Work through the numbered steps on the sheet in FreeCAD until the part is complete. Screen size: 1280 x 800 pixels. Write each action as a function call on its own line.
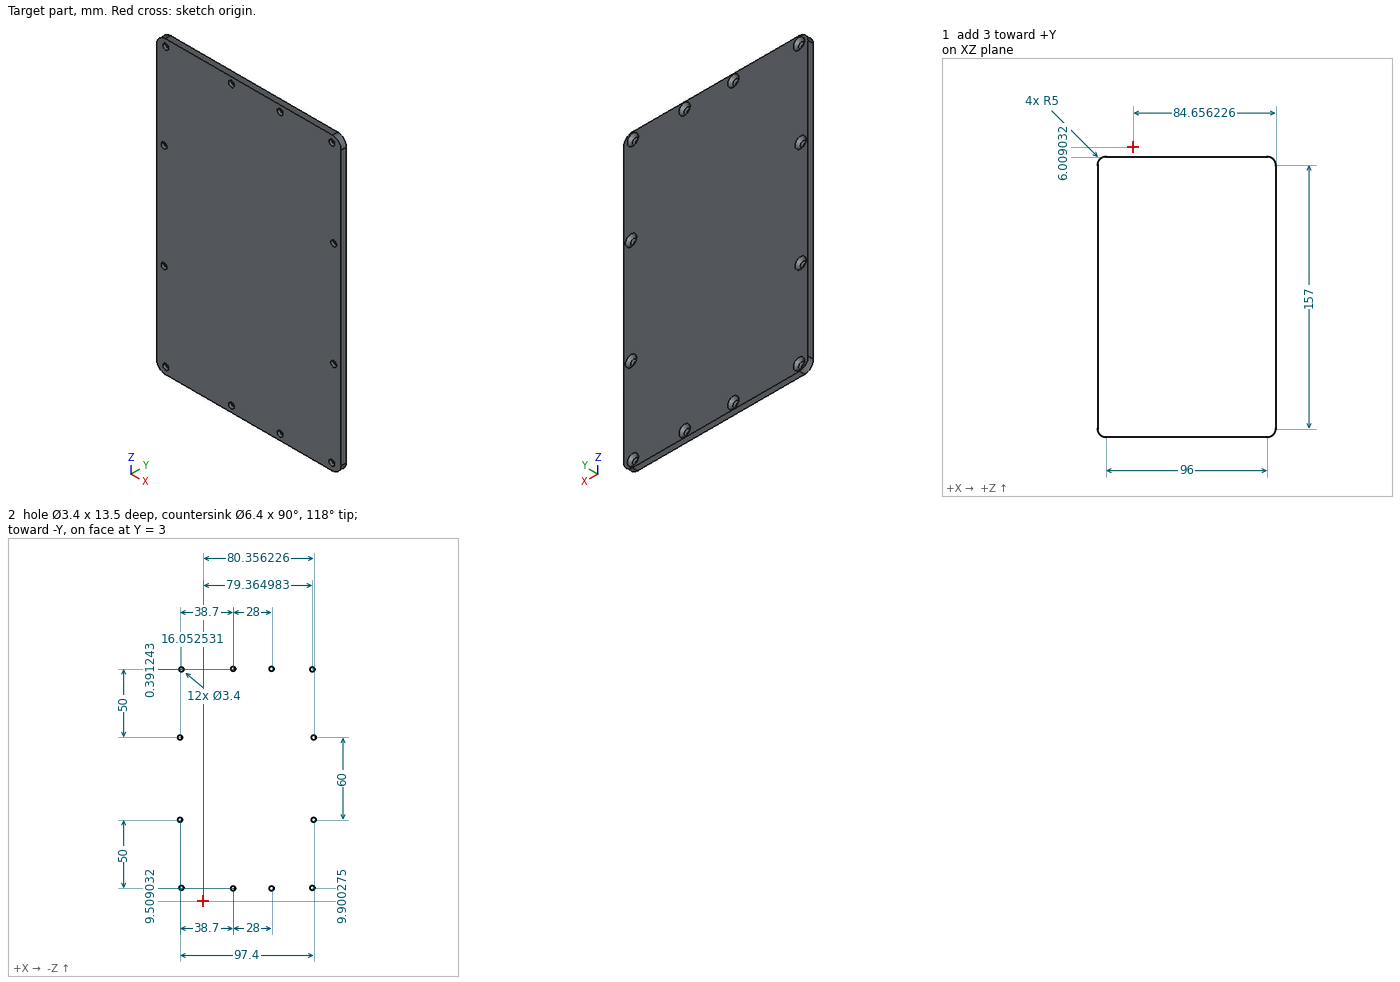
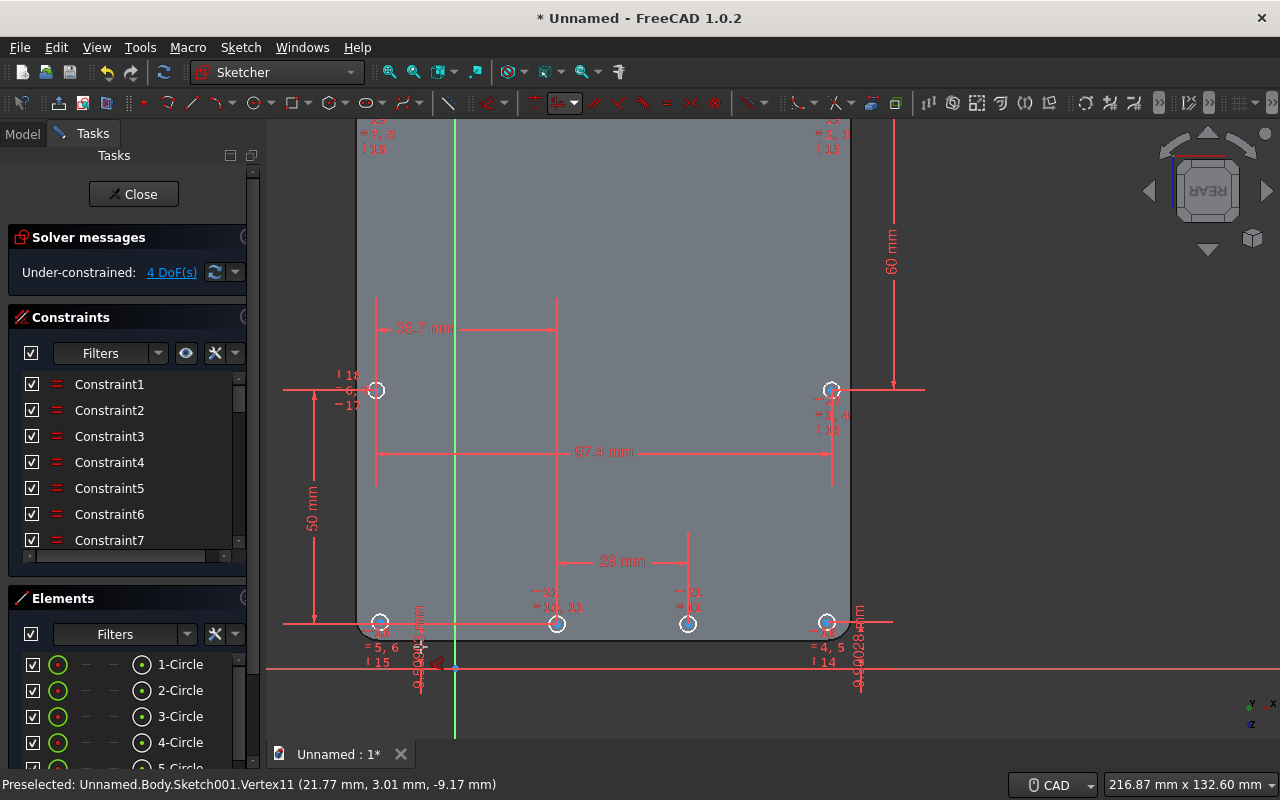
scroll(827, 624, down, 3)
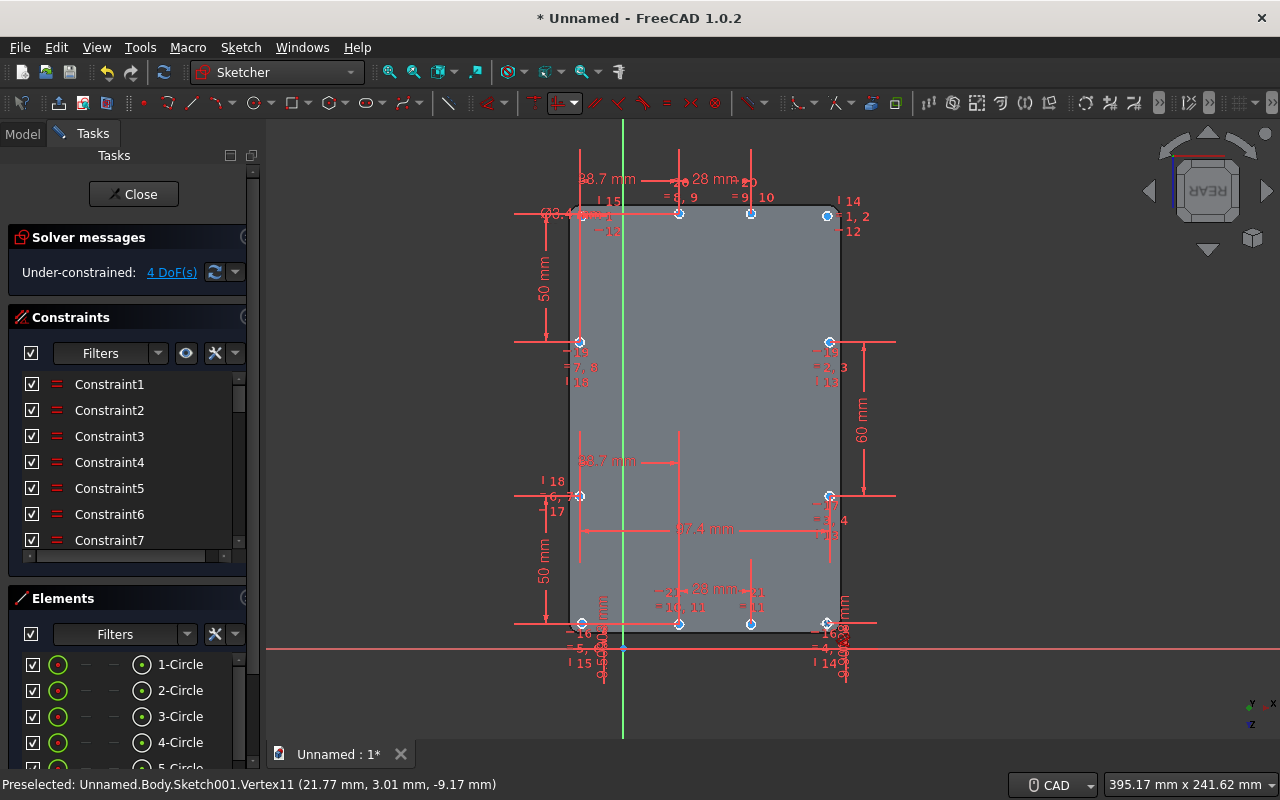
click(582, 216)
click(603, 683)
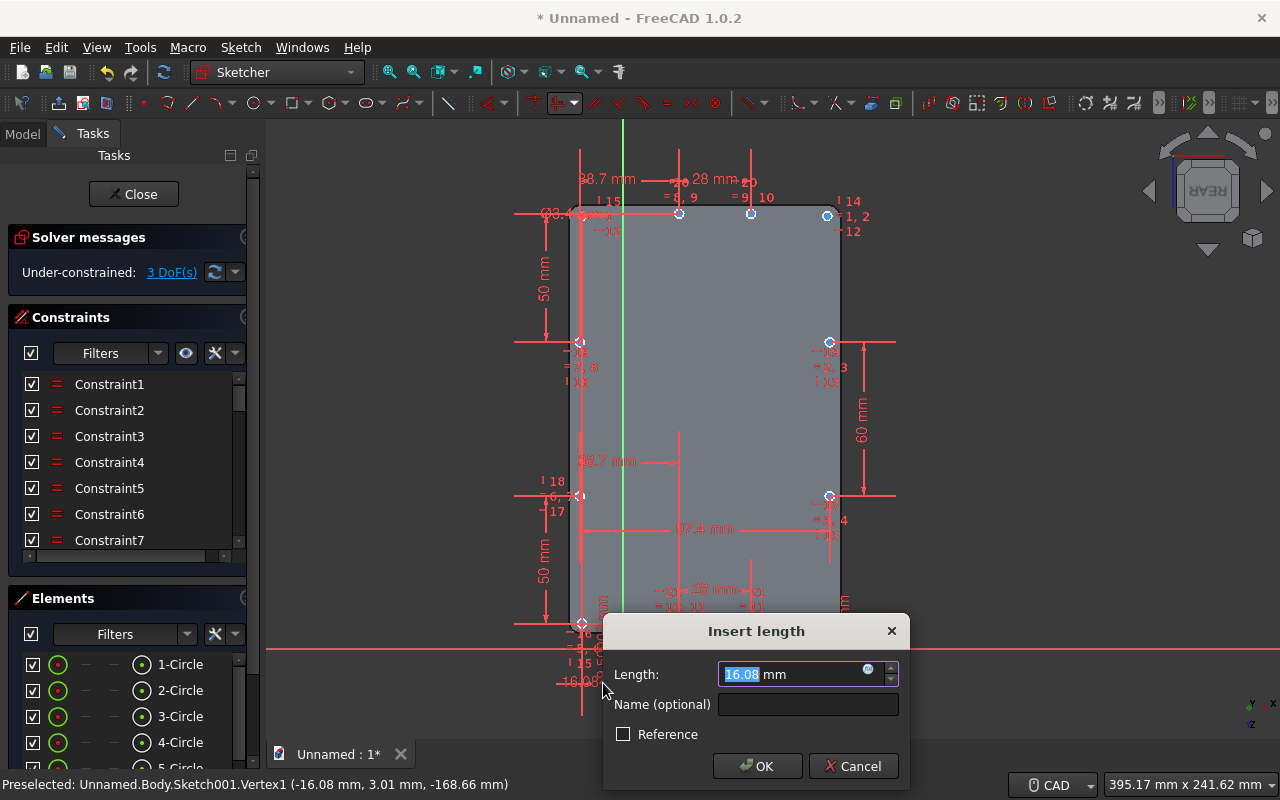
text(16.052531)
key(Return)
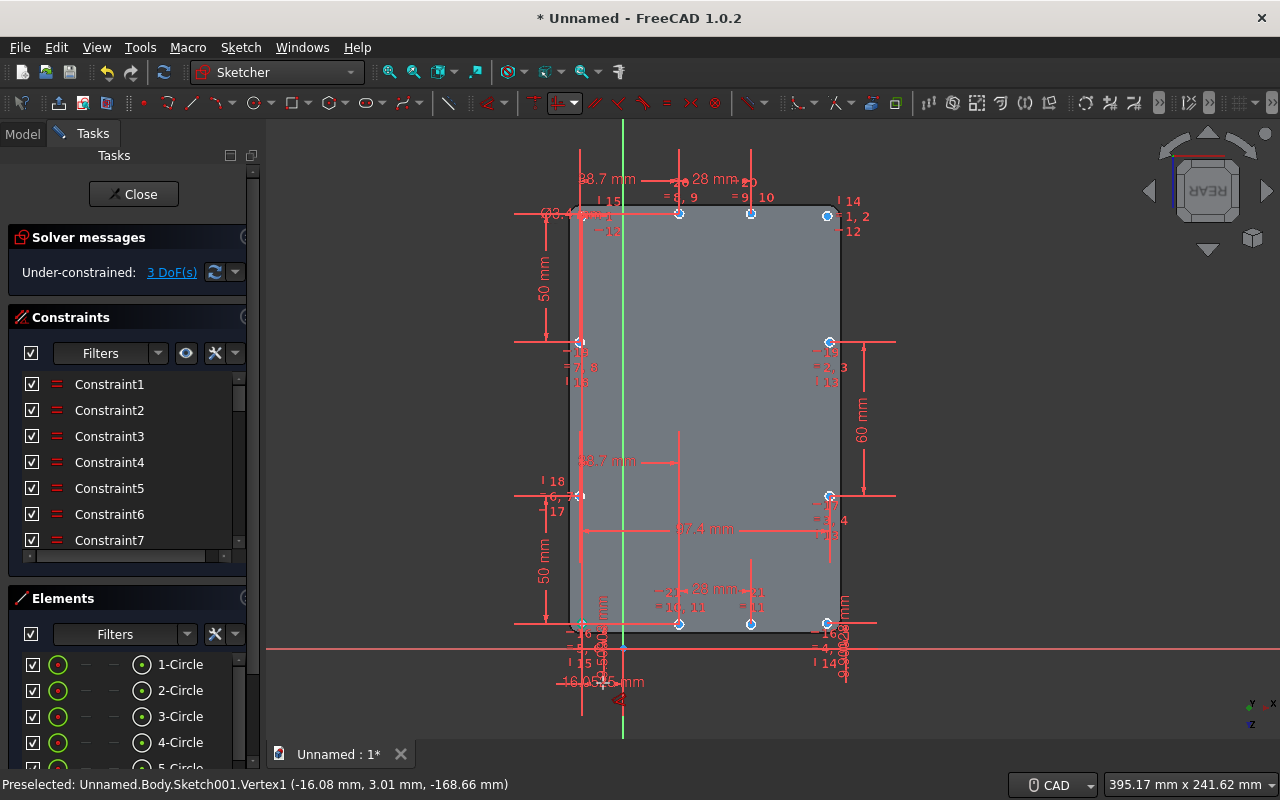
click(827, 216)
click(725, 683)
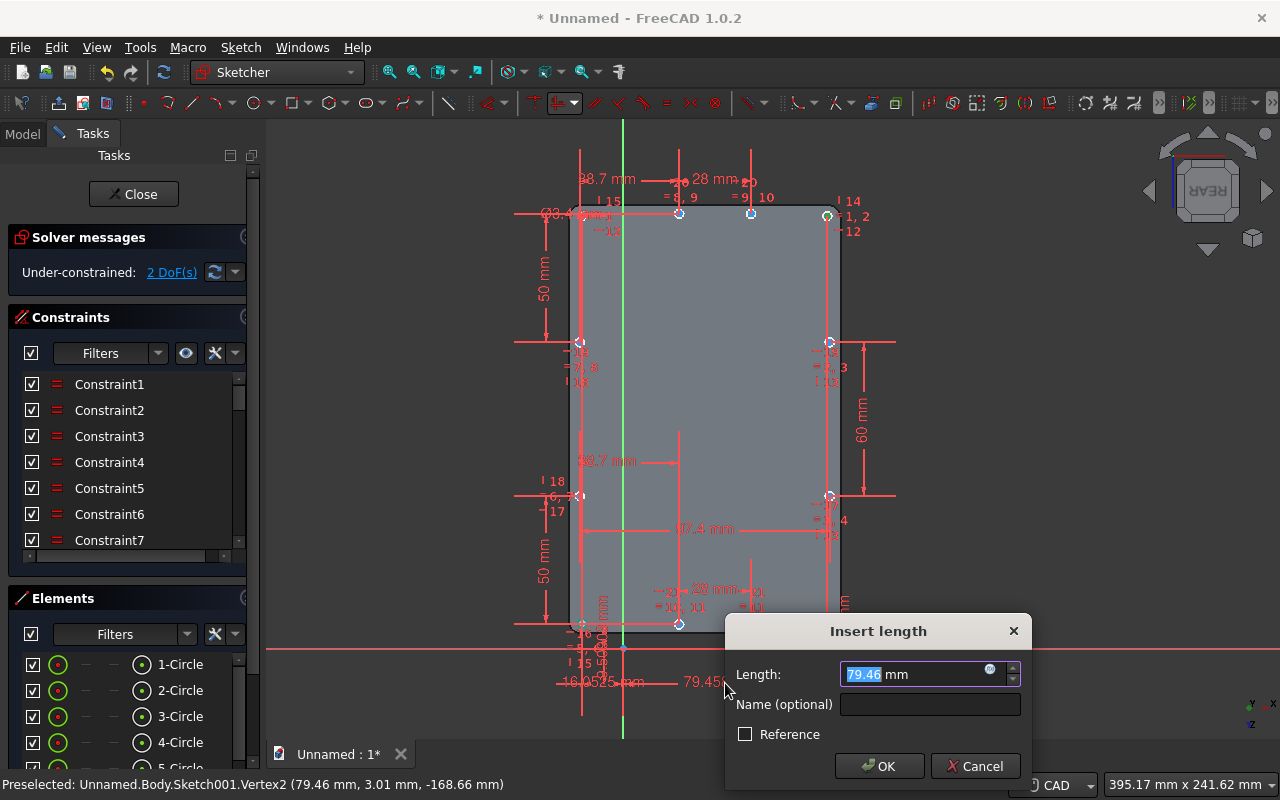
text(79.364983)
key(Return)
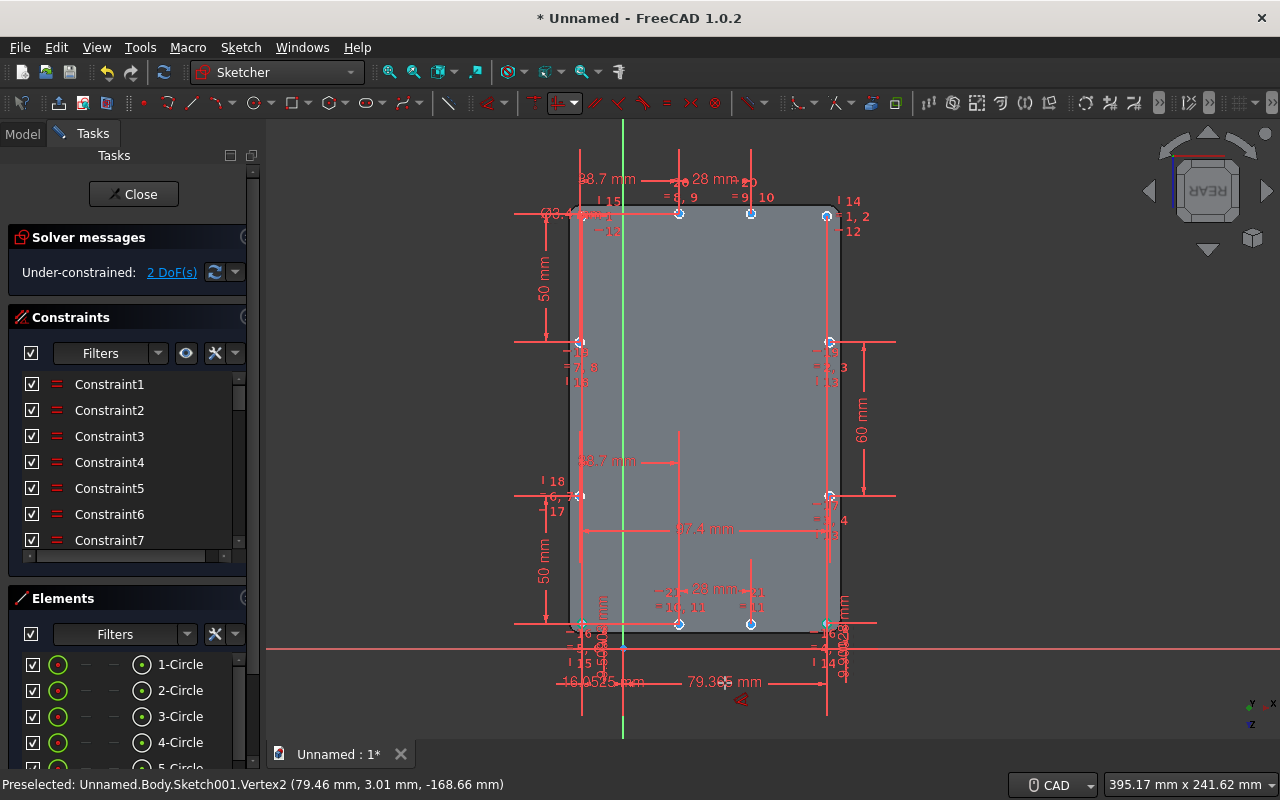
click(830, 342)
click(799, 683)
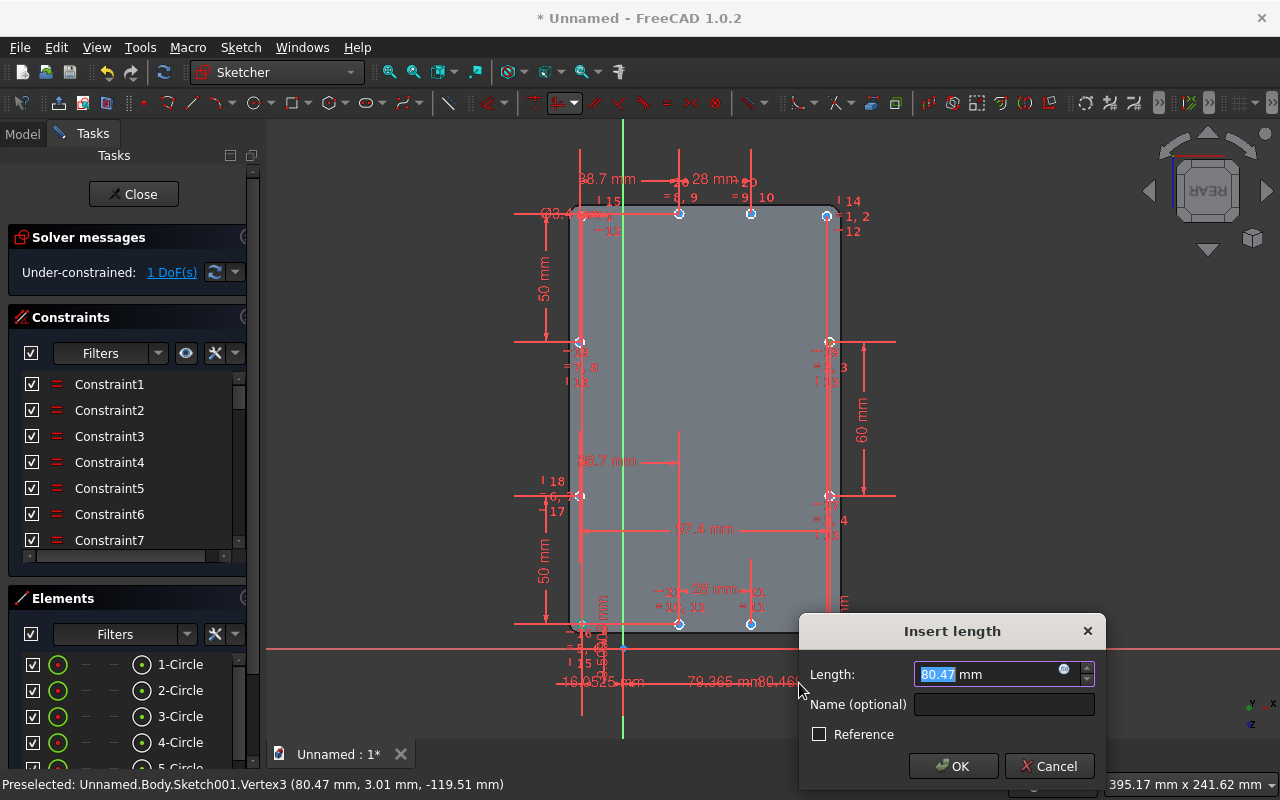
text(80.356226)
key(Return)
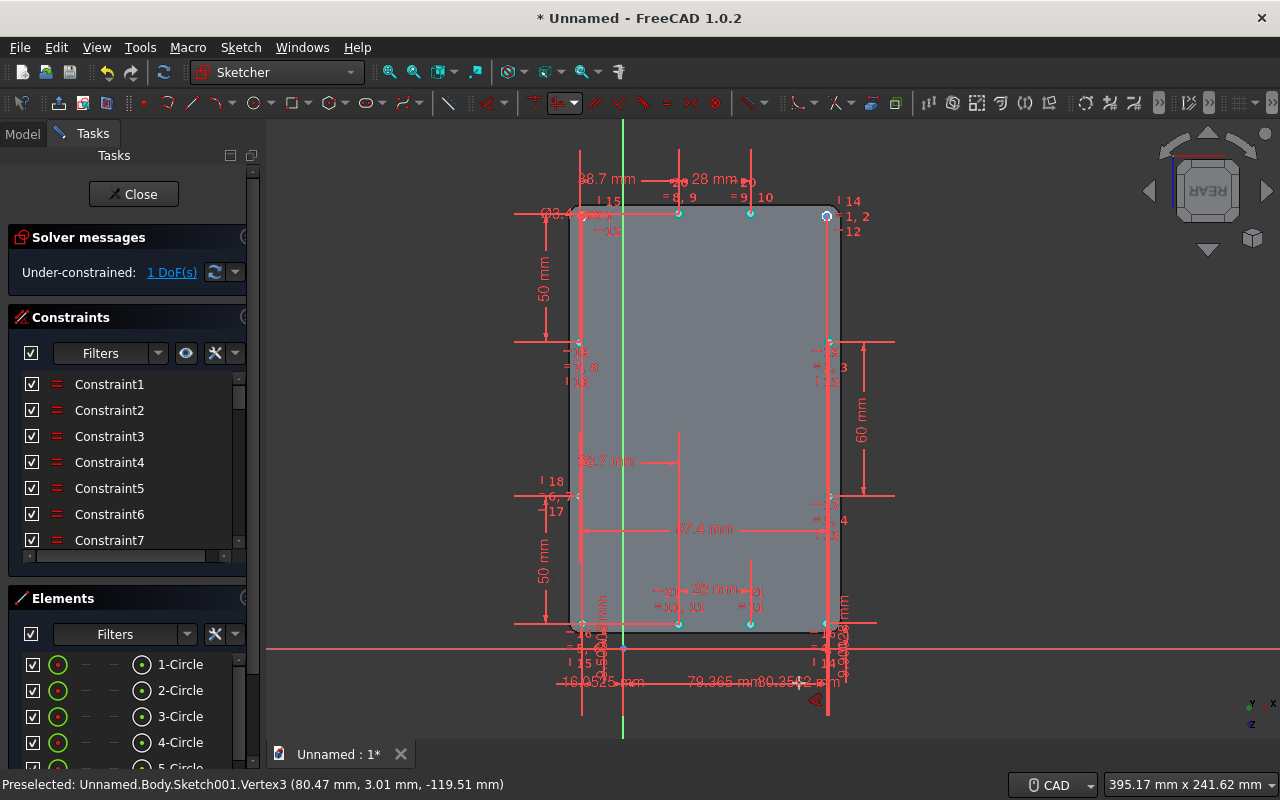
scroll(582, 216, up, 19)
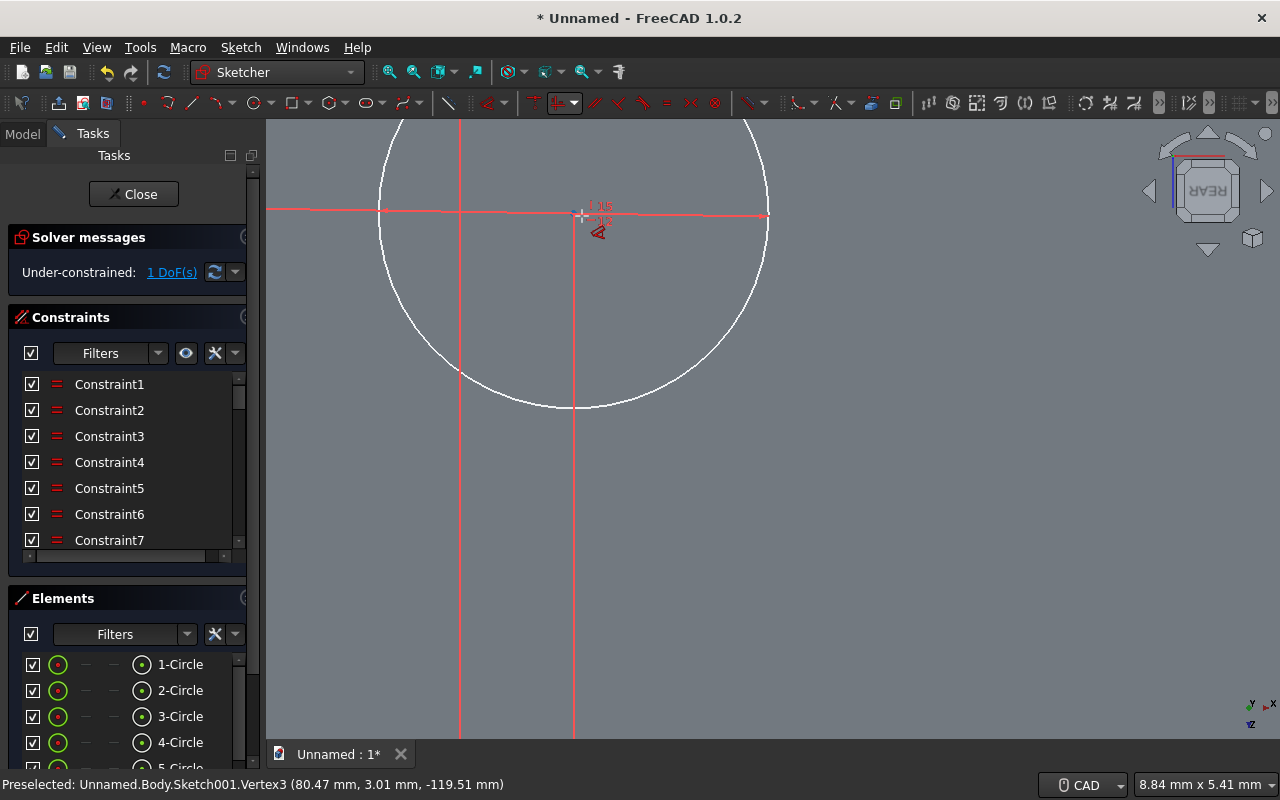
click(574, 214)